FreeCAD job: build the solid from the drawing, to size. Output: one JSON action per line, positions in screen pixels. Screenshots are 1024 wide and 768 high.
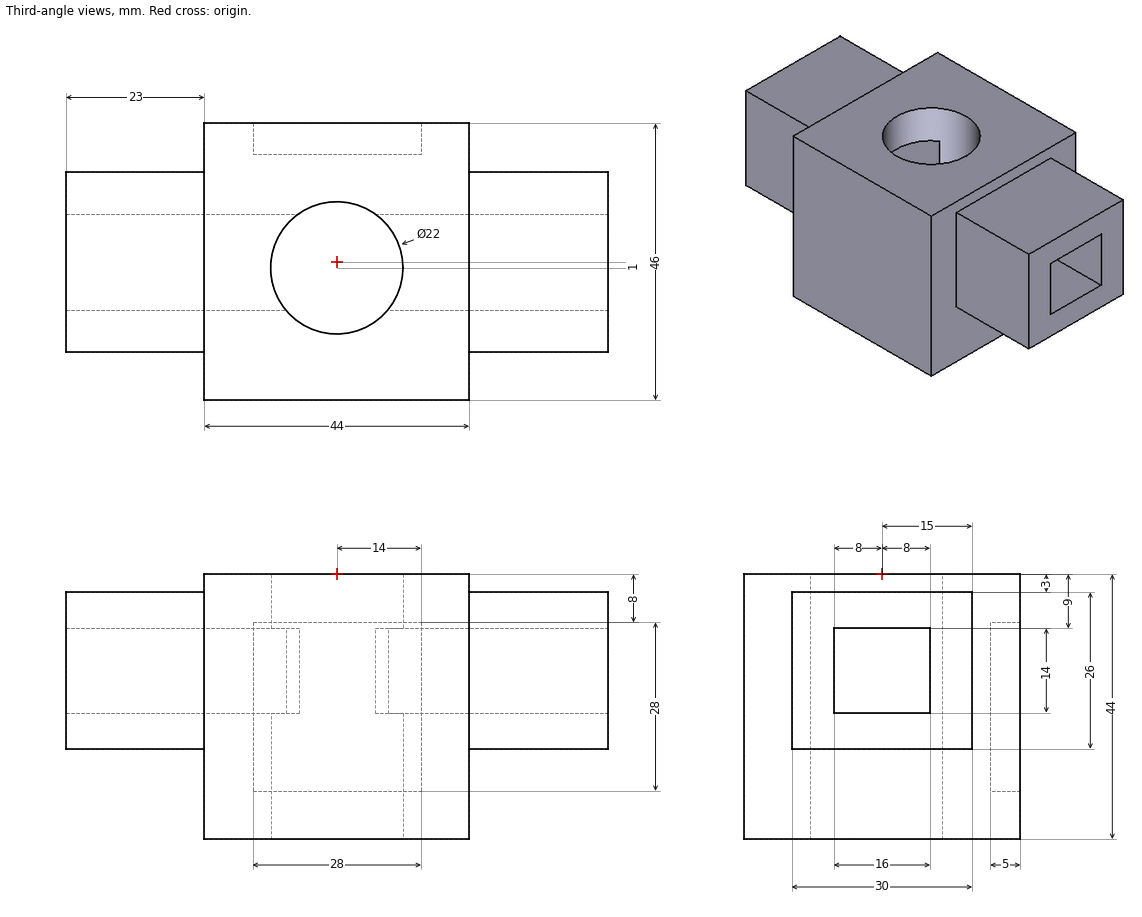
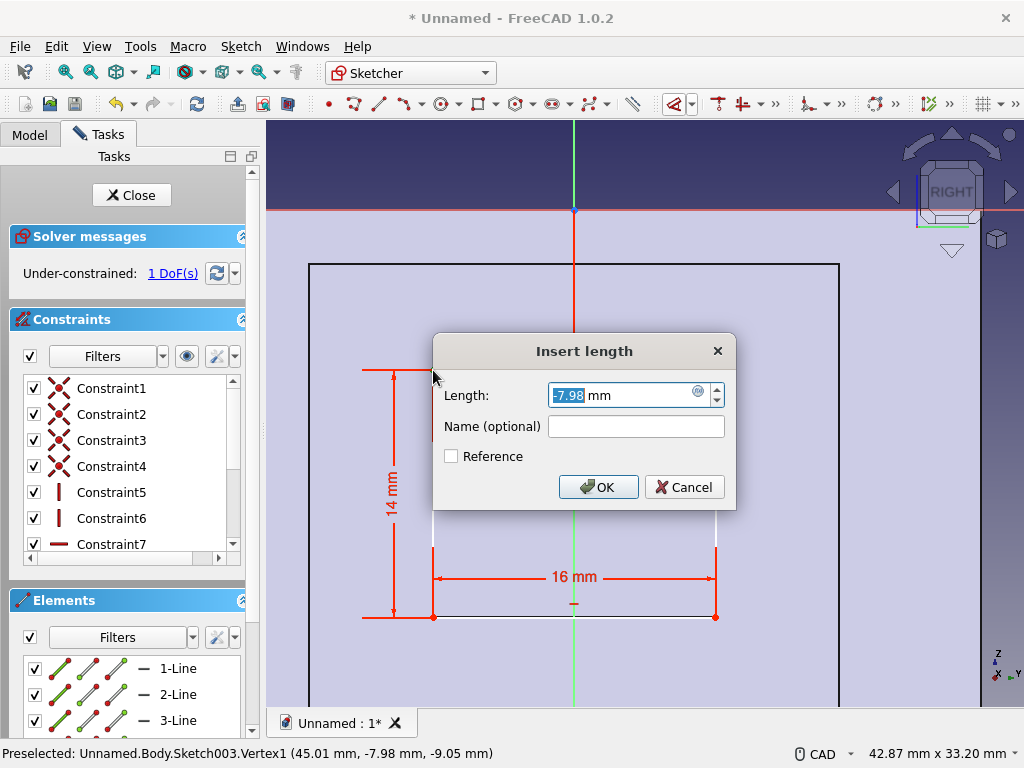
{"action": "type", "text": "-8"}
{"action": "key", "text": "Return"}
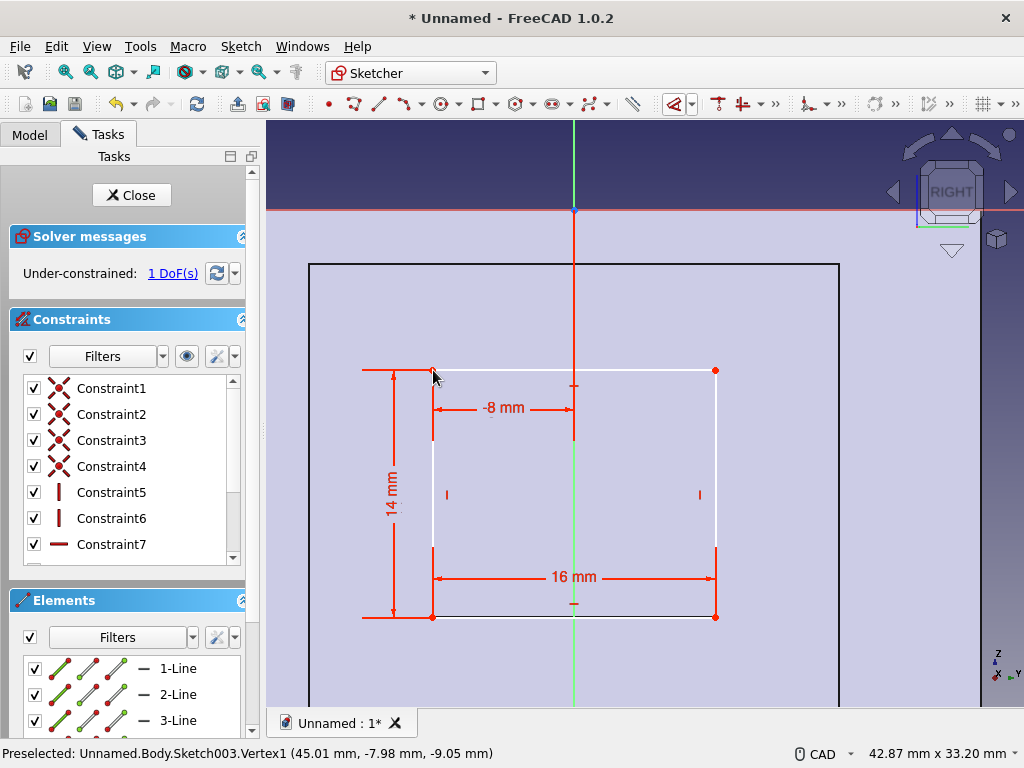
{"action": "left_click", "coordinate": [433, 370]}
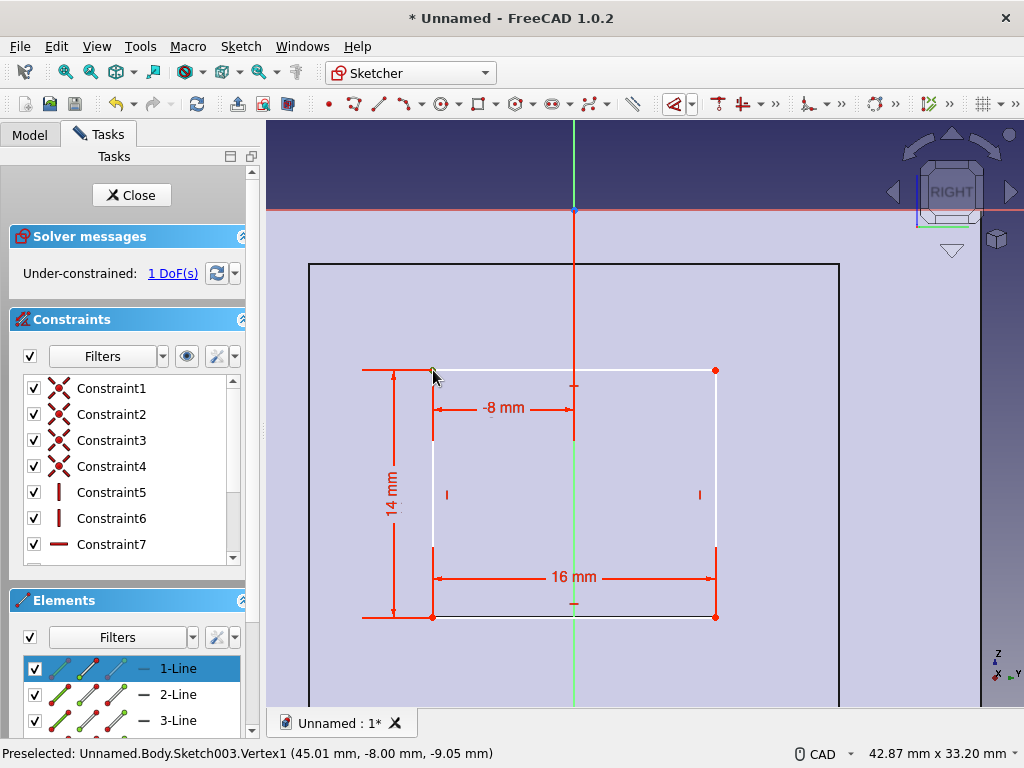
{"action": "key", "text": "i"}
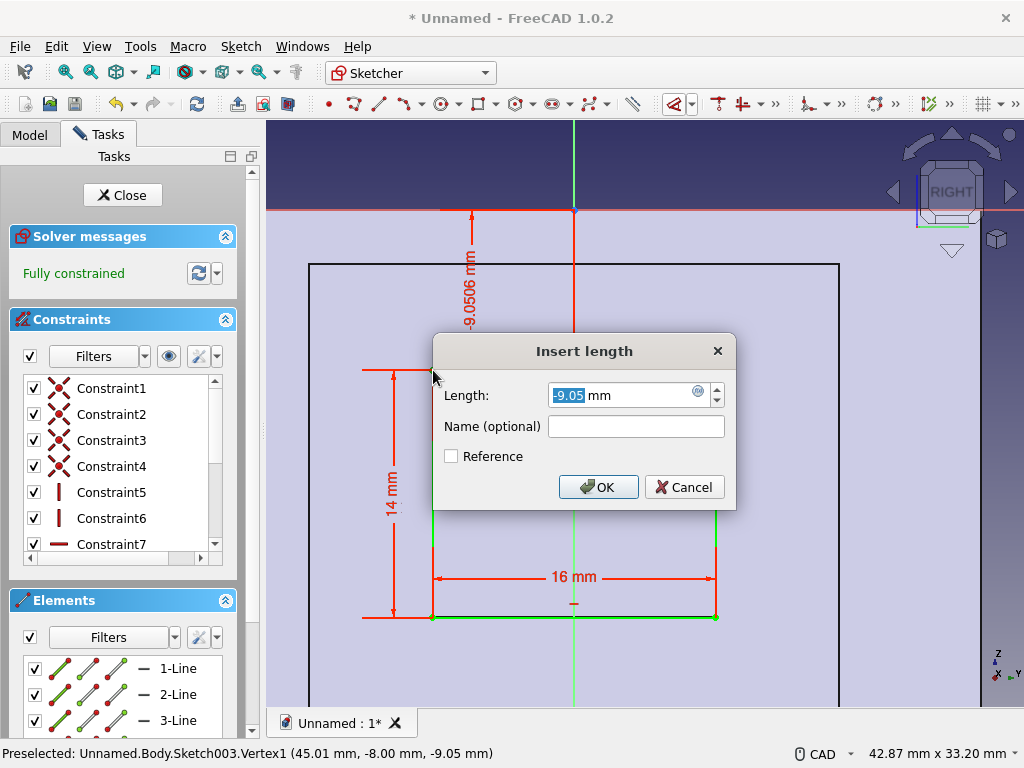
{"action": "type", "text": "-9"}
{"action": "key", "text": "Return"}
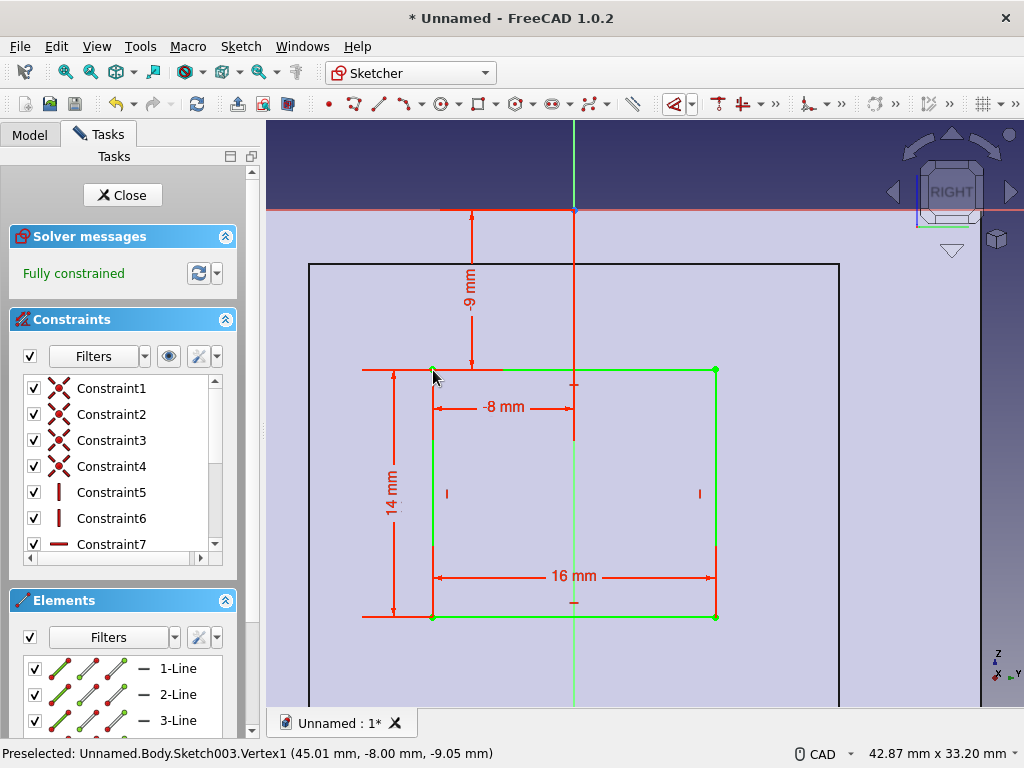
{"action": "left_click", "coordinate": [123, 195]}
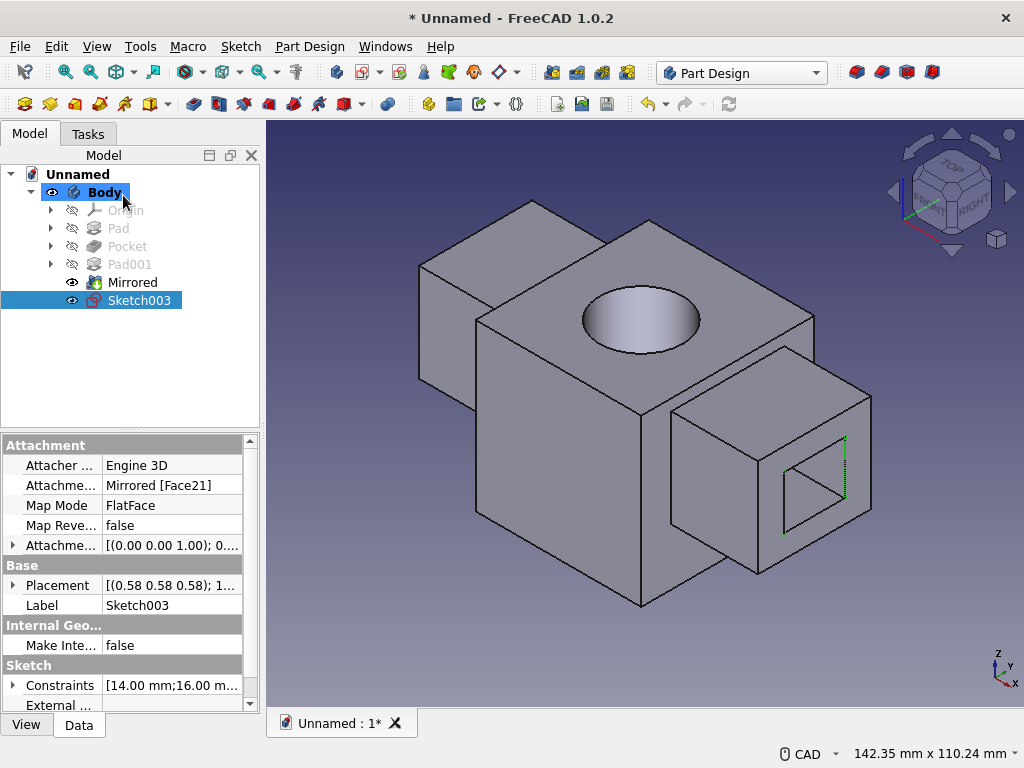
{"action": "left_click", "coordinate": [194, 104]}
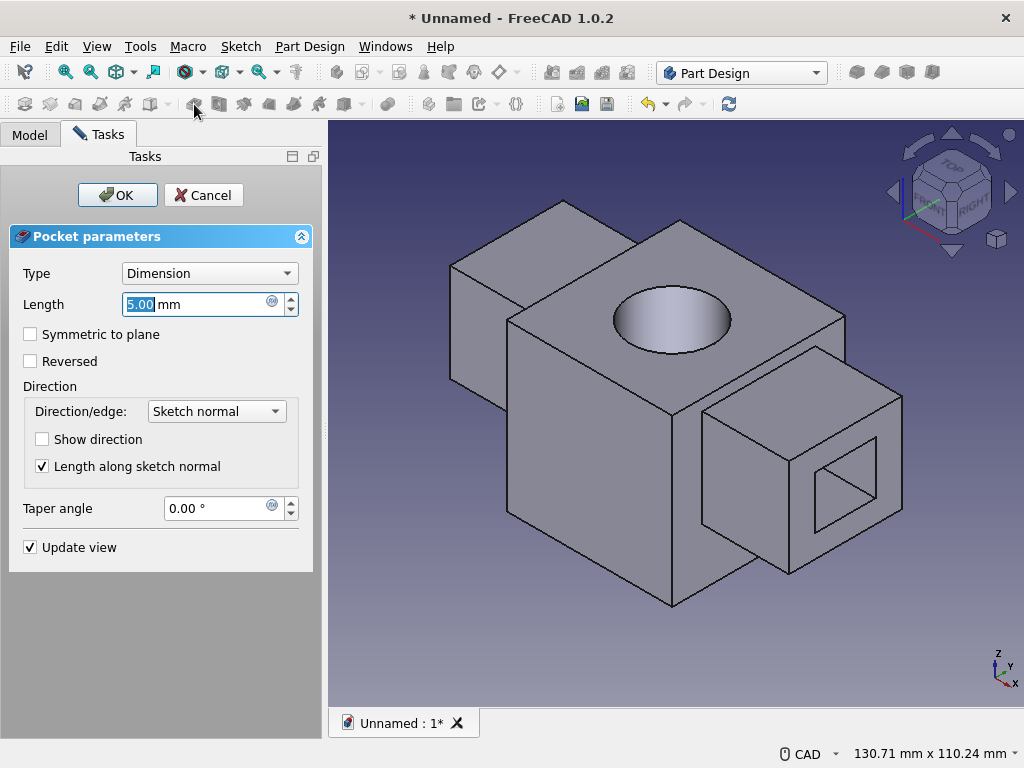
{"action": "left_click", "coordinate": [210, 274]}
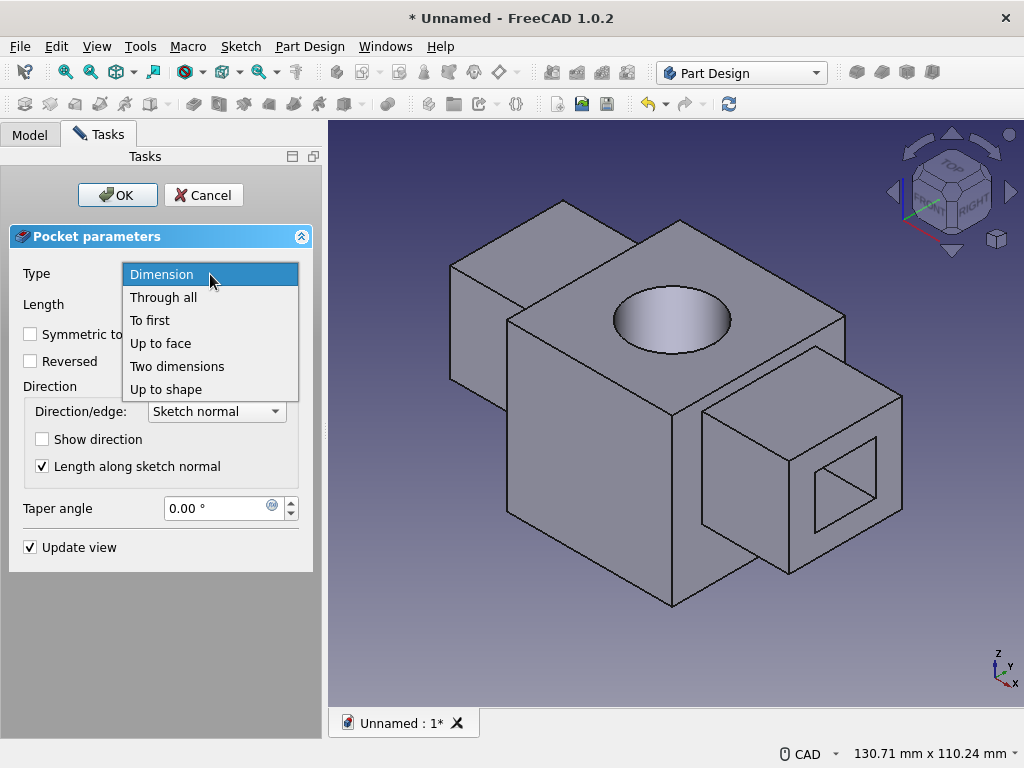
{"action": "left_click", "coordinate": [208, 298]}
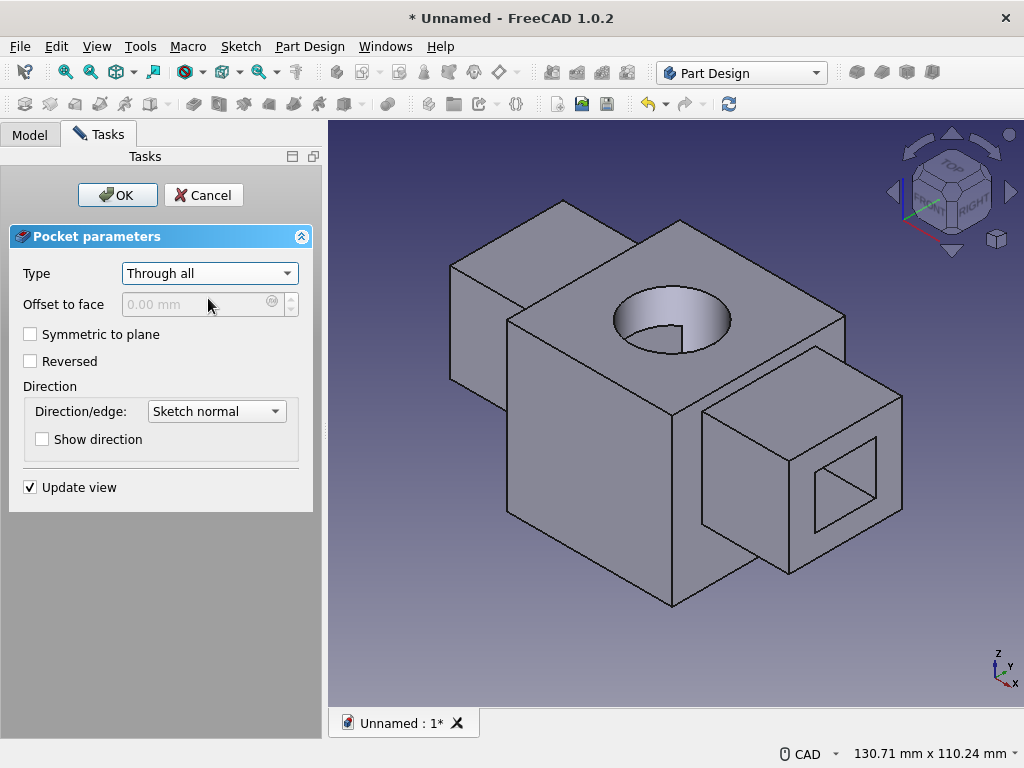
{"action": "left_click", "coordinate": [118, 195]}